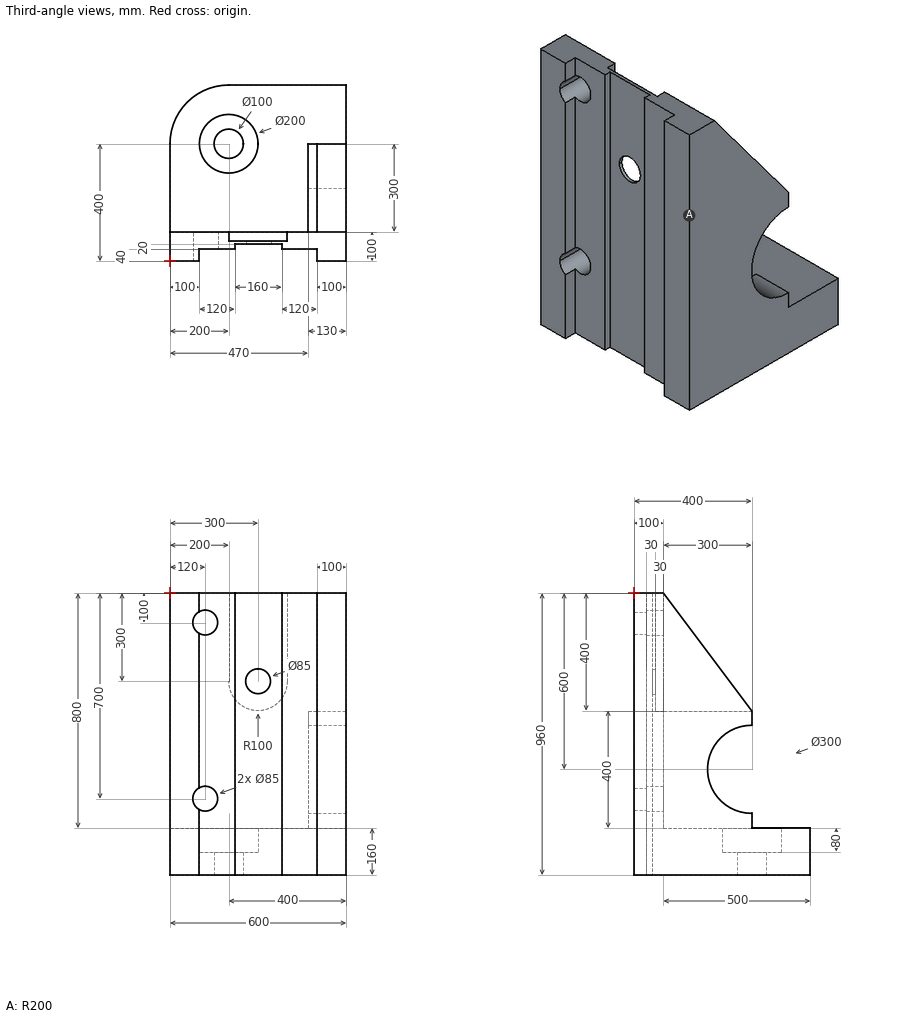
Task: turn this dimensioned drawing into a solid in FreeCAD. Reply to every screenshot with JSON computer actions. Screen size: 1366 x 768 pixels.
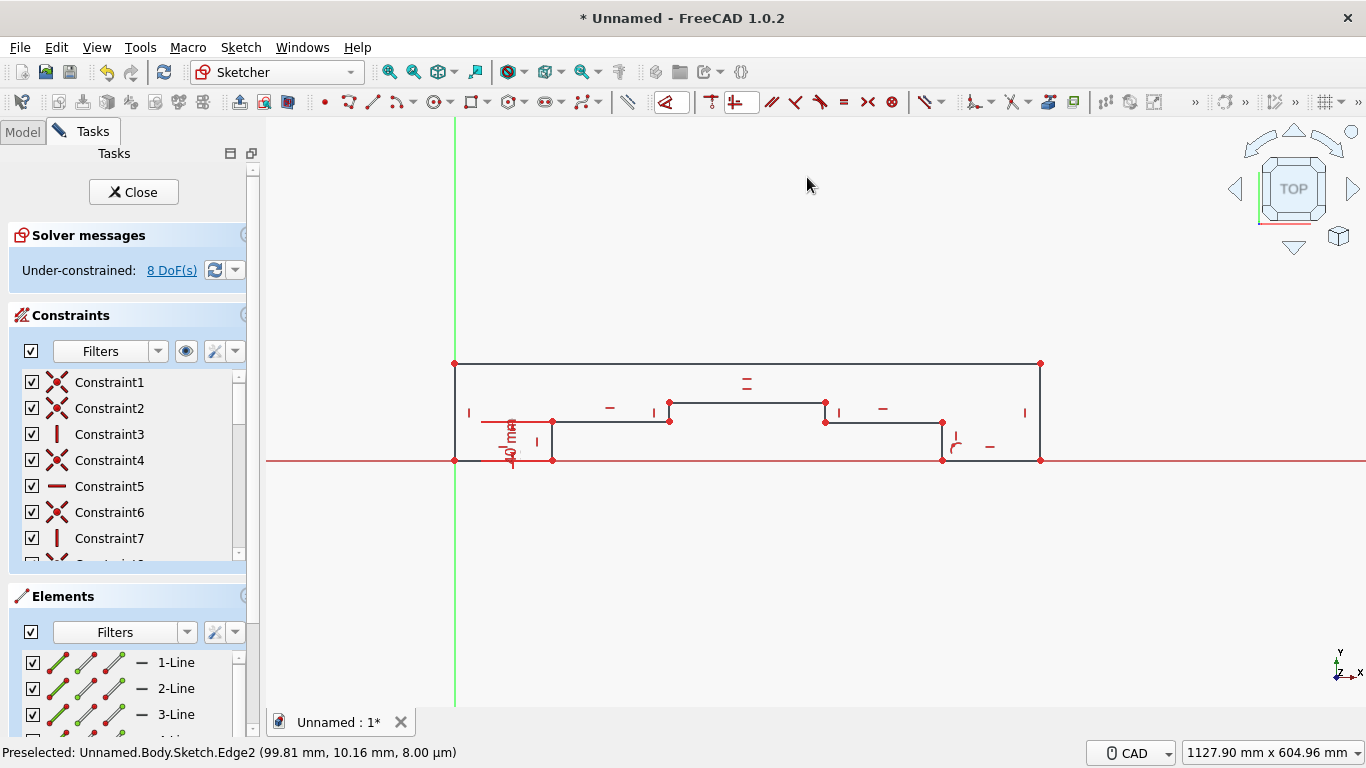
{"action": "scroll", "coordinate": [669, 412], "scroll_direction": "up", "scroll_amount": 4}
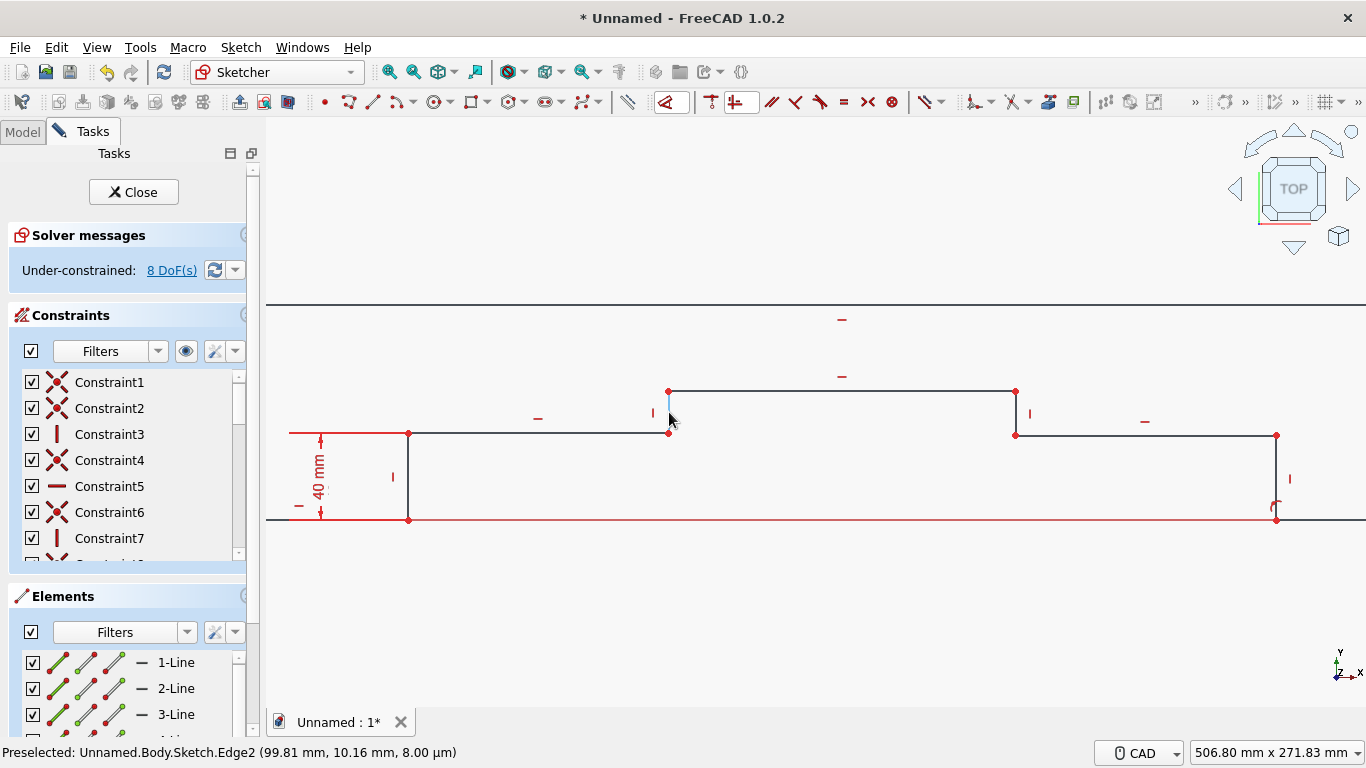
{"action": "left_click", "coordinate": [669, 412]}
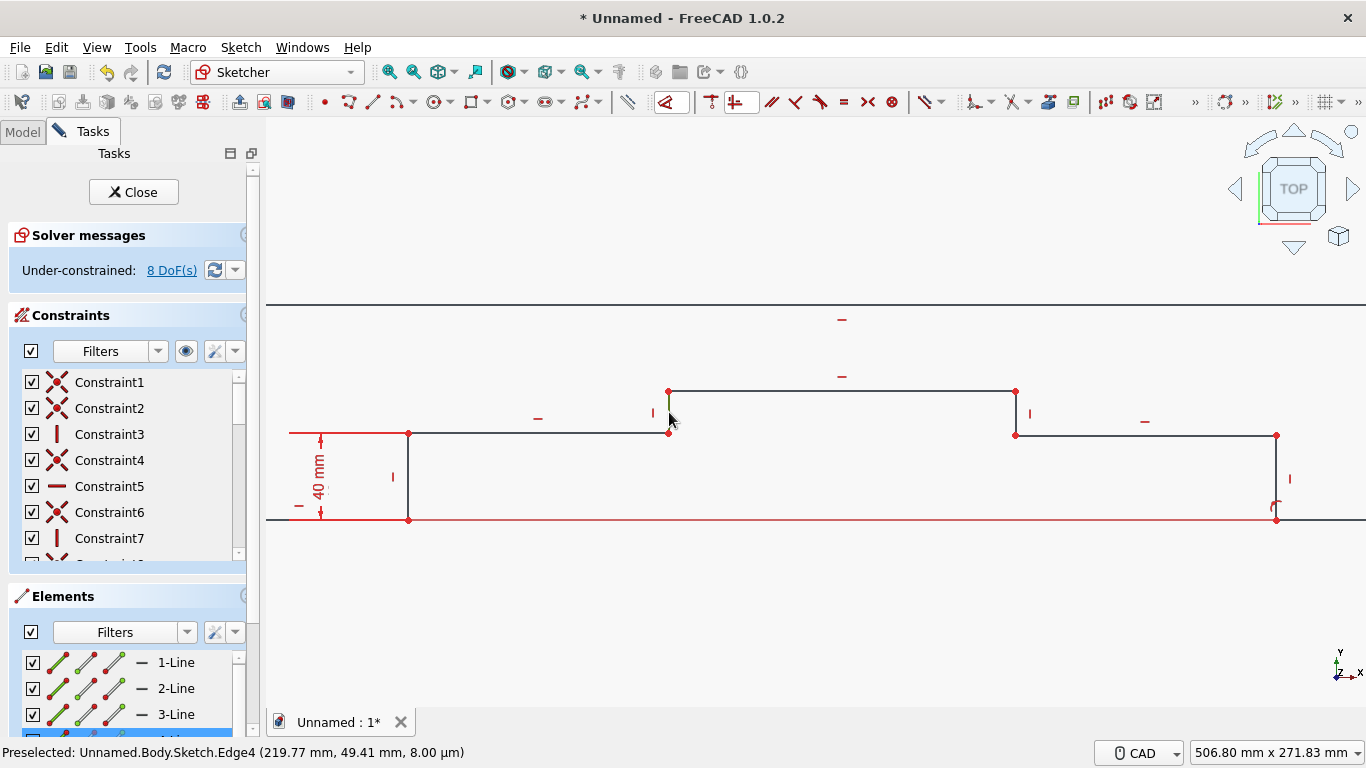
{"action": "left_click", "coordinate": [684, 102]}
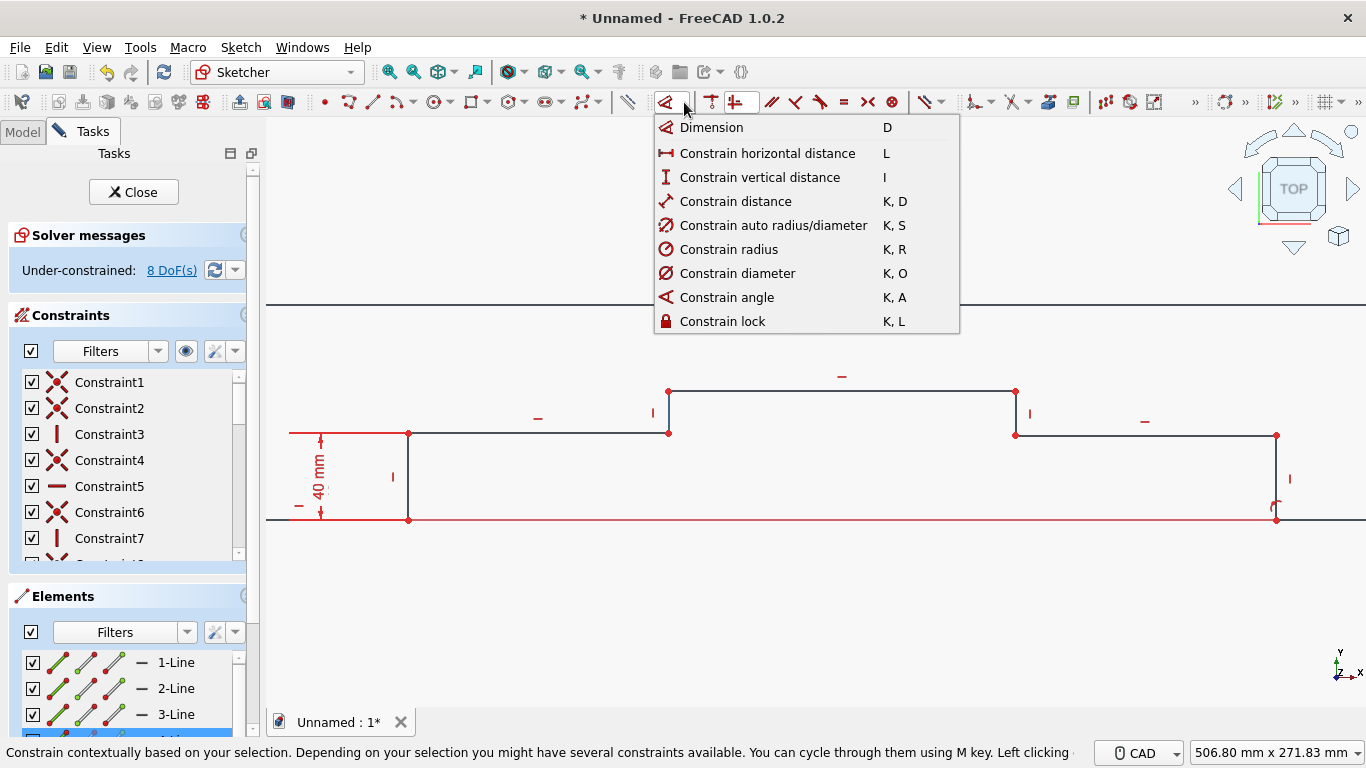
{"action": "left_click", "coordinate": [807, 177]}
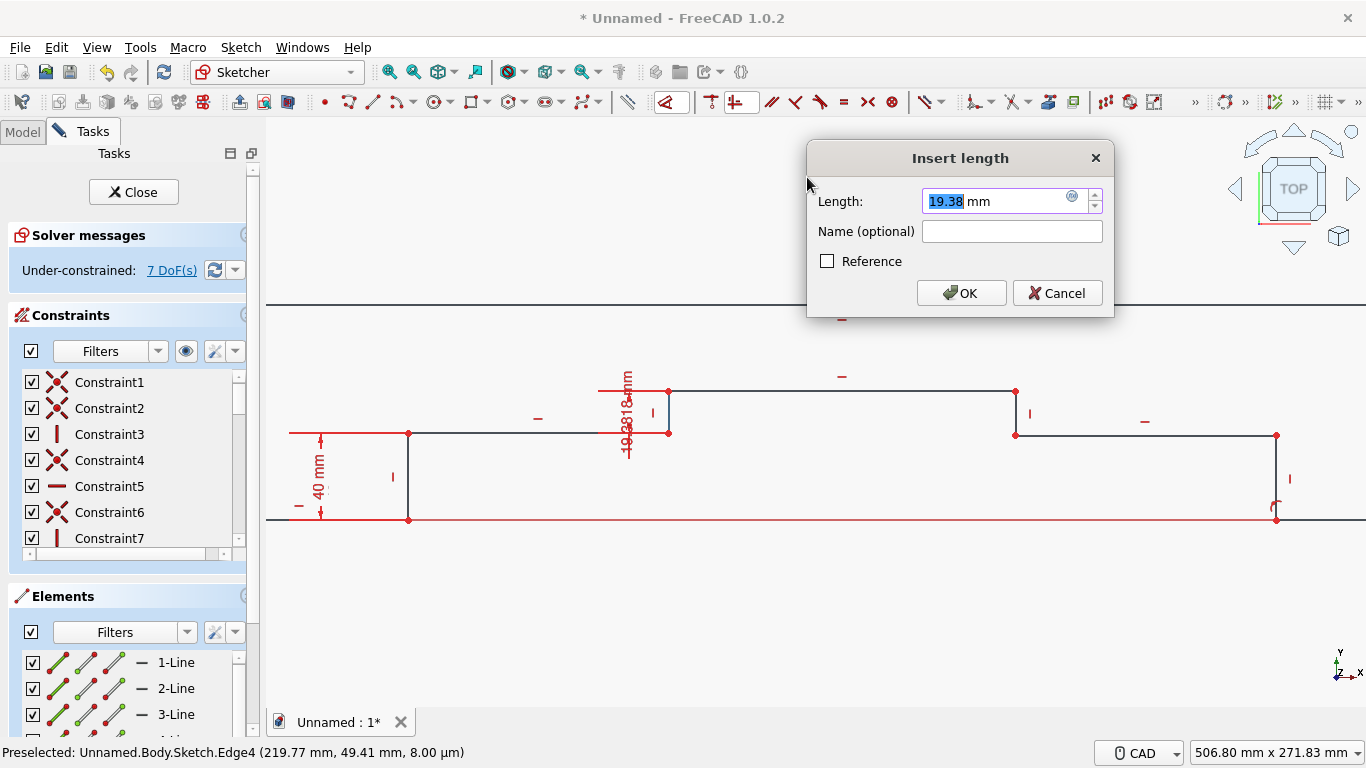
{"action": "type", "text": "20"}
{"action": "key", "text": "Return"}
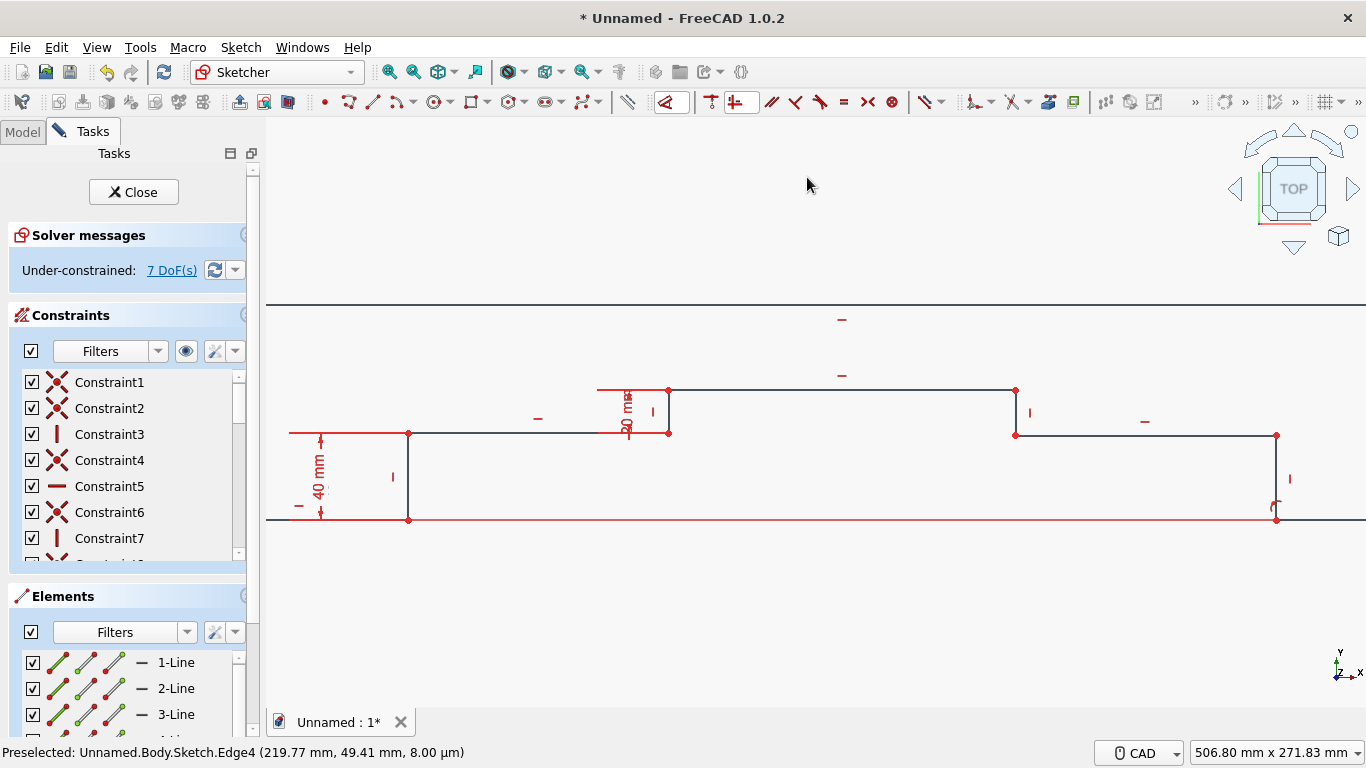
{"action": "left_click", "coordinate": [1016, 404]}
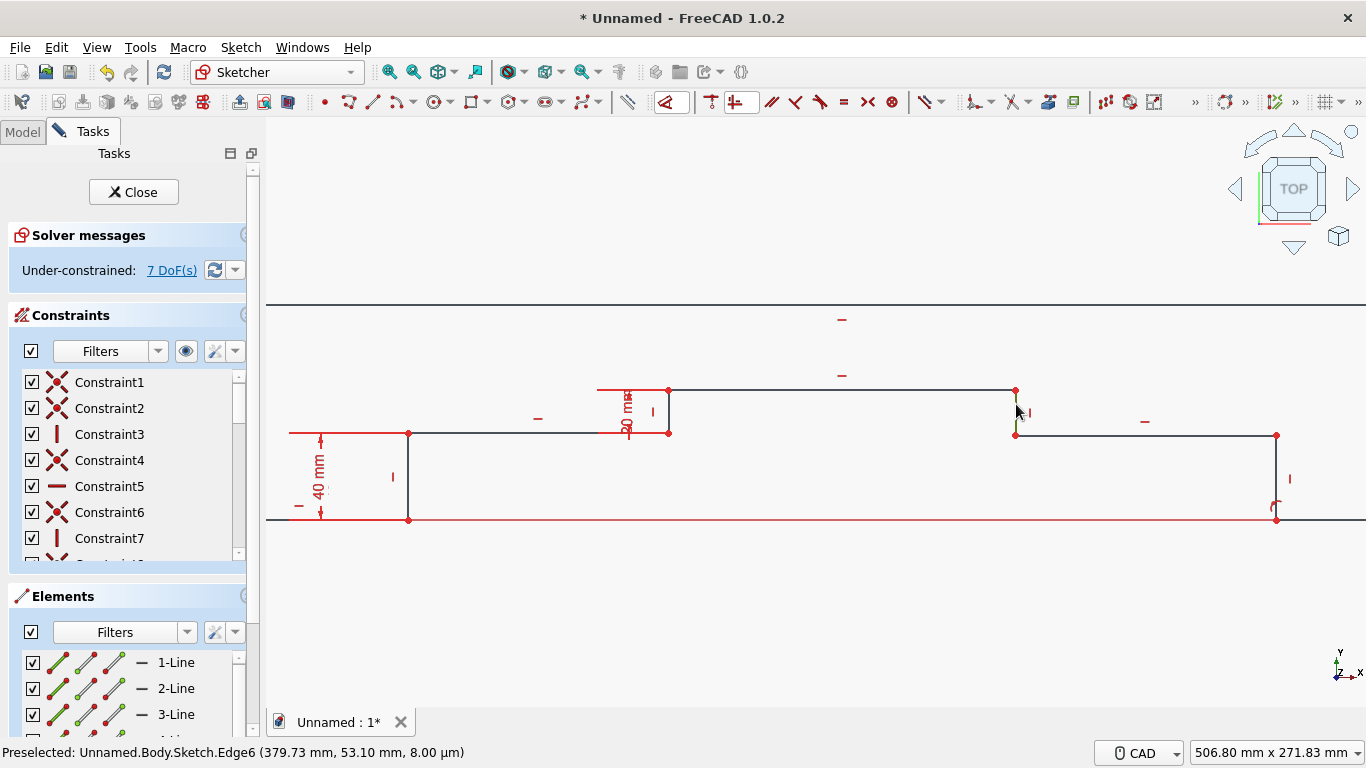
{"action": "key", "text": "i"}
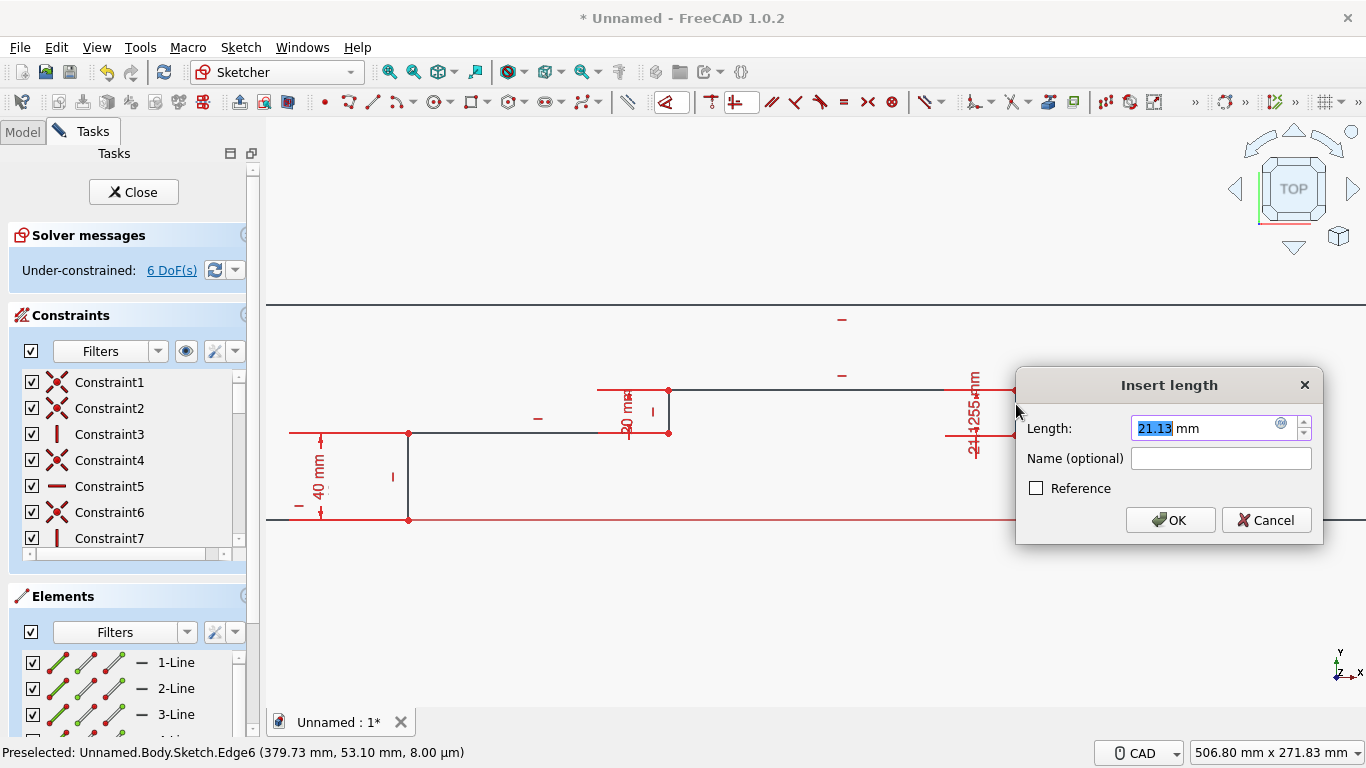
{"action": "type", "text": "20"}
{"action": "key", "text": "Return"}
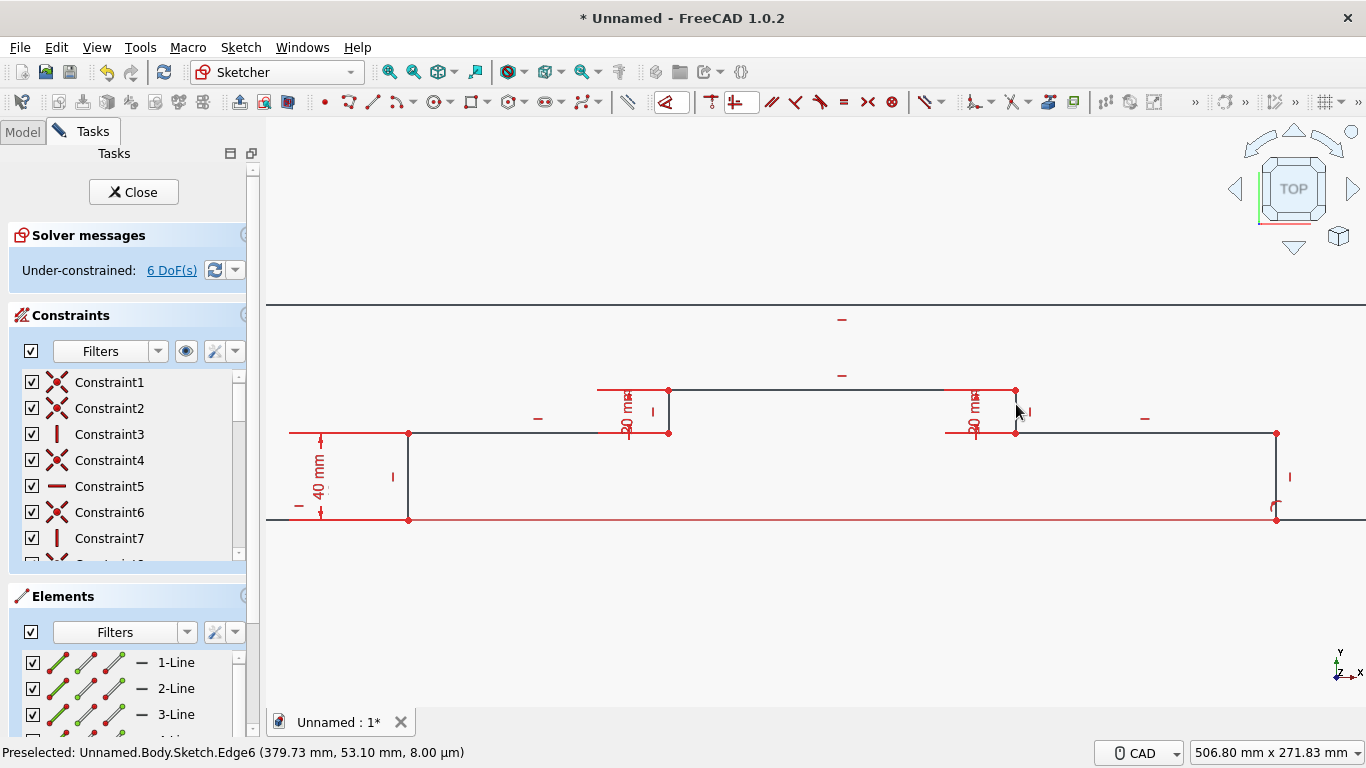
{"action": "left_click", "coordinate": [343, 520]}